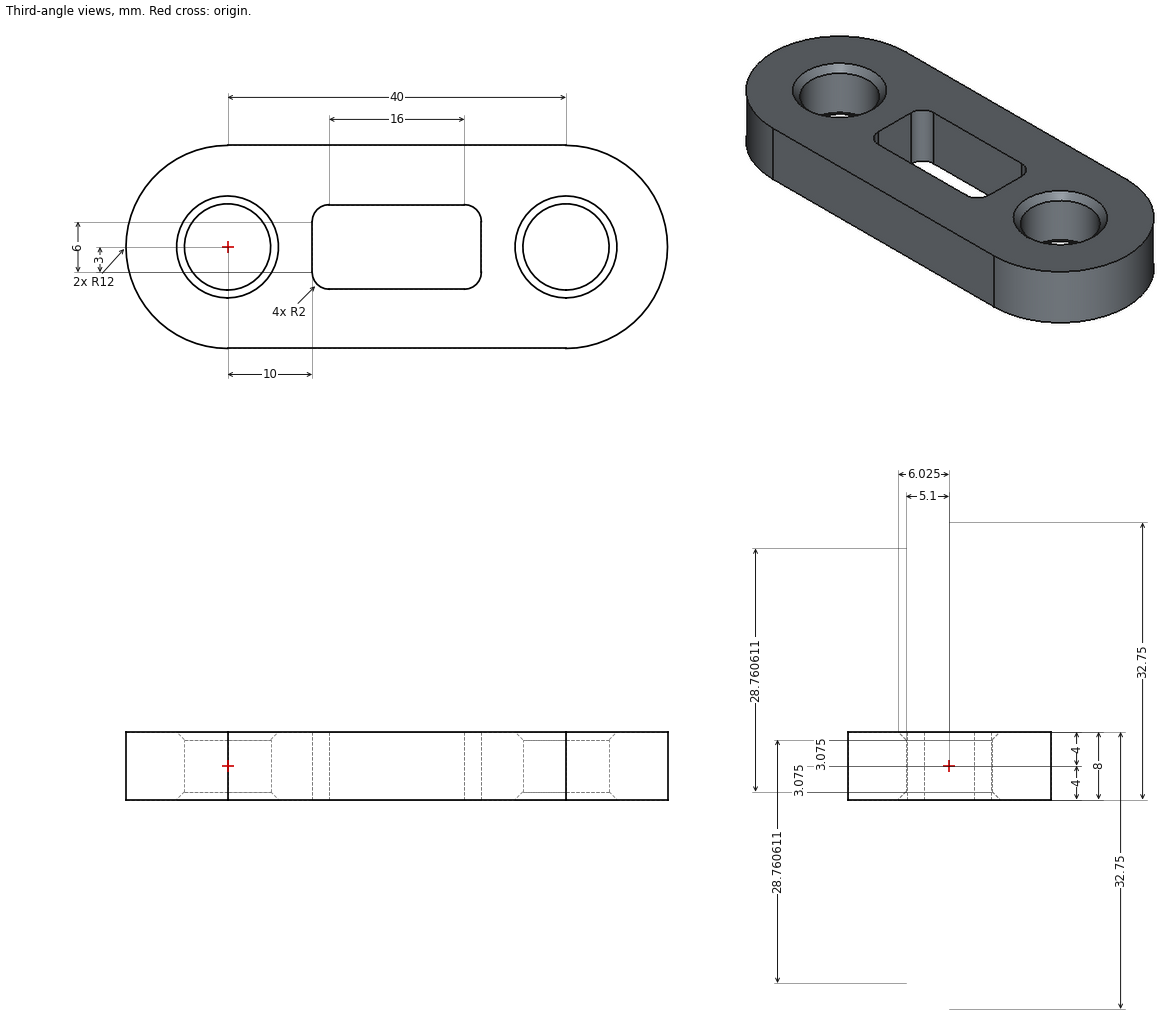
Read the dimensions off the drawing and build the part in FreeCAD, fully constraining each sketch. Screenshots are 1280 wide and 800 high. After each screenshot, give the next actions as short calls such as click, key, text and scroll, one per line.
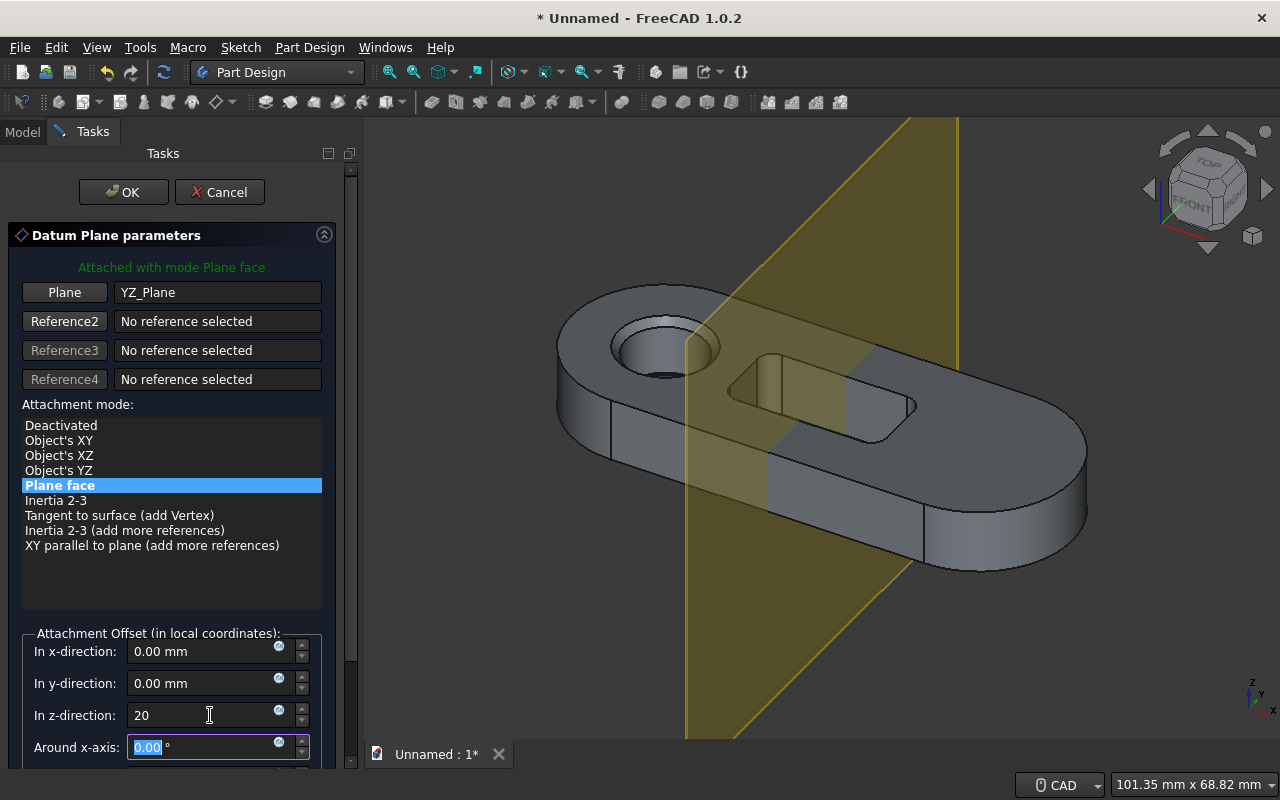
click(124, 192)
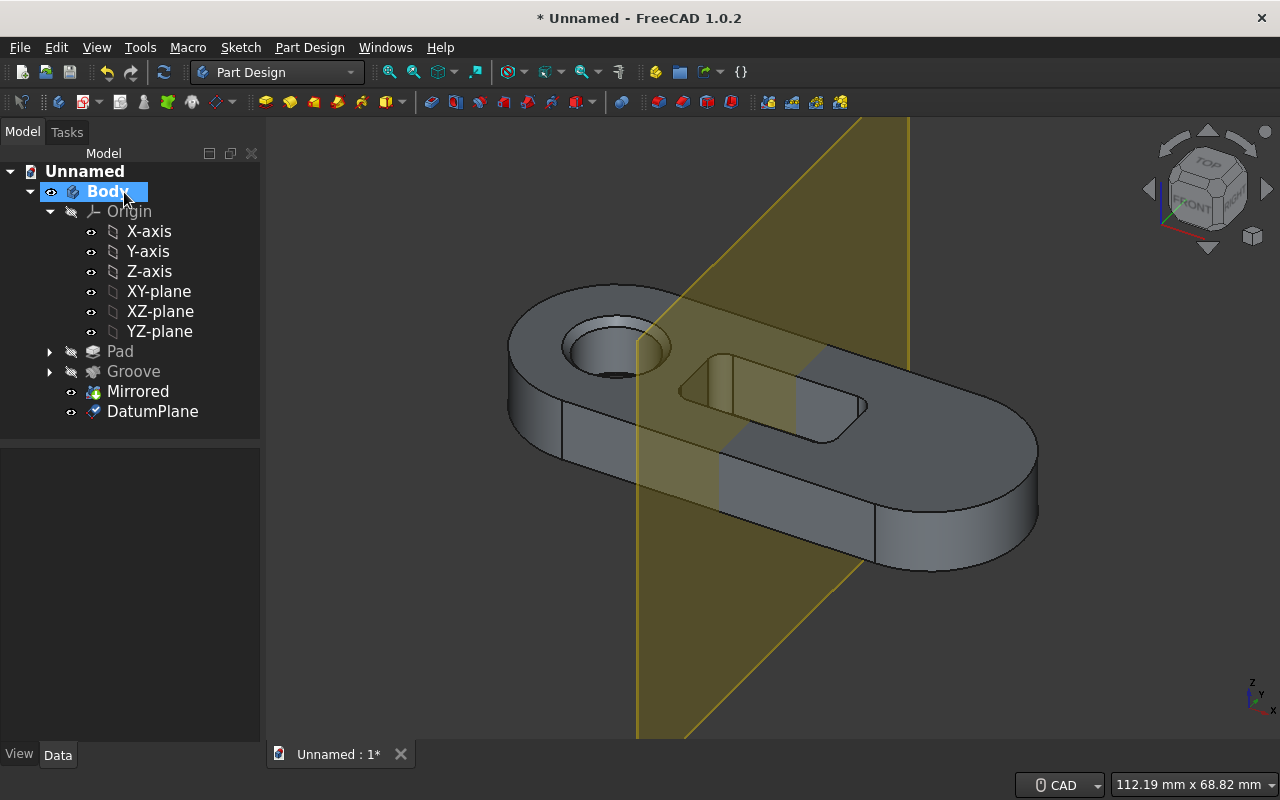
click(116, 372)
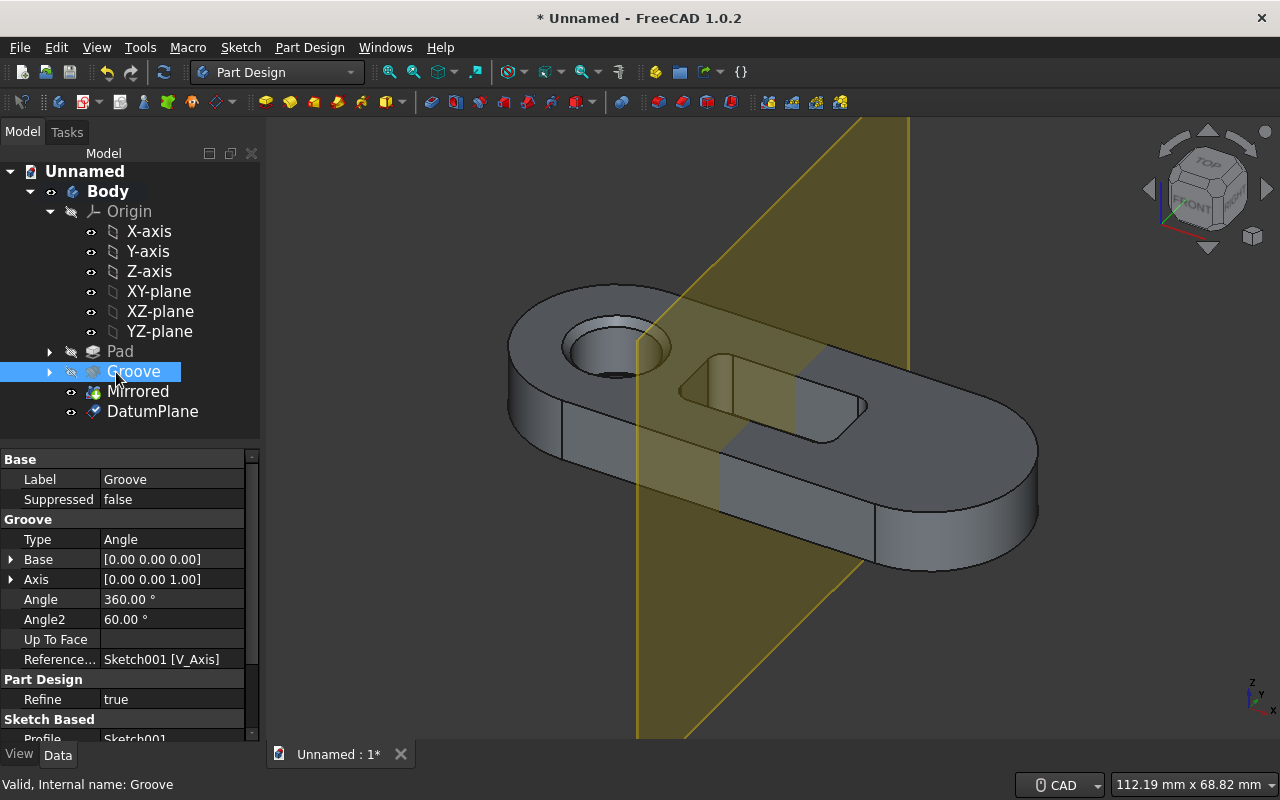
click(768, 102)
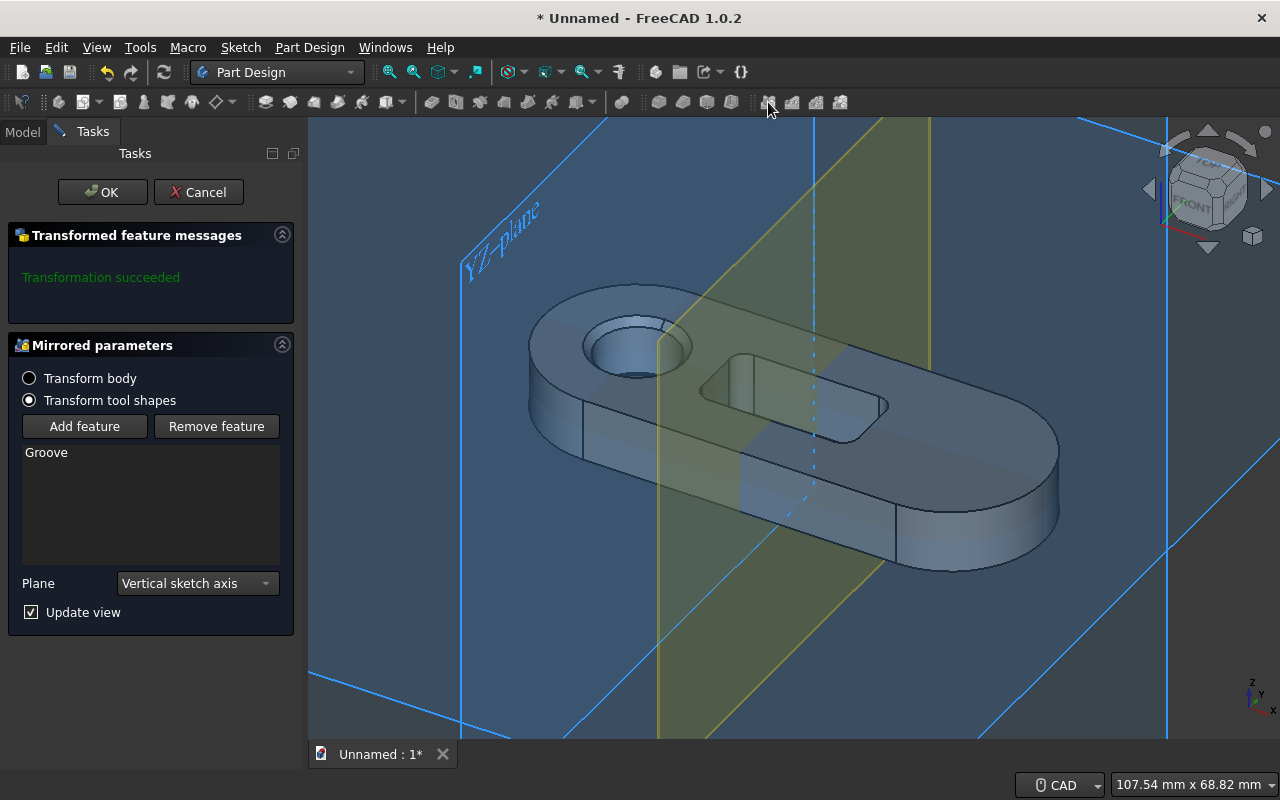
click(198, 584)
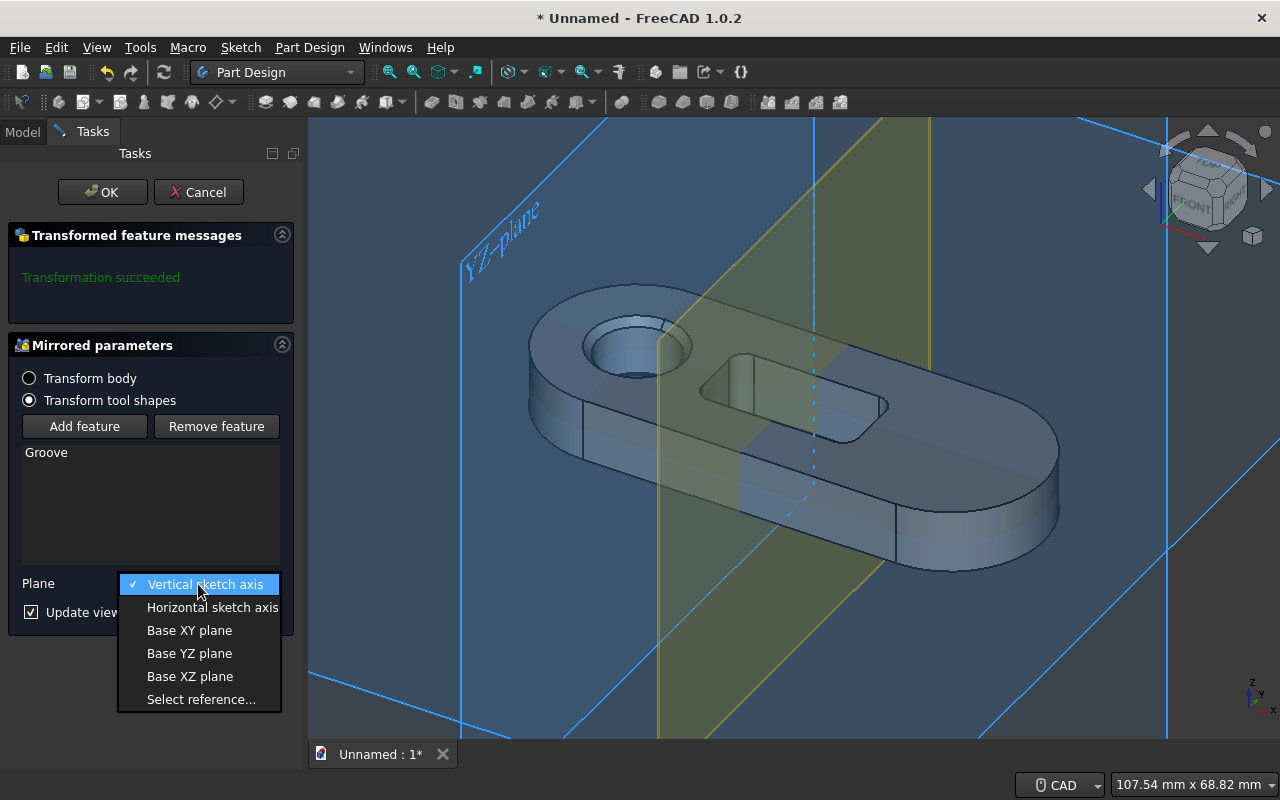
click(198, 700)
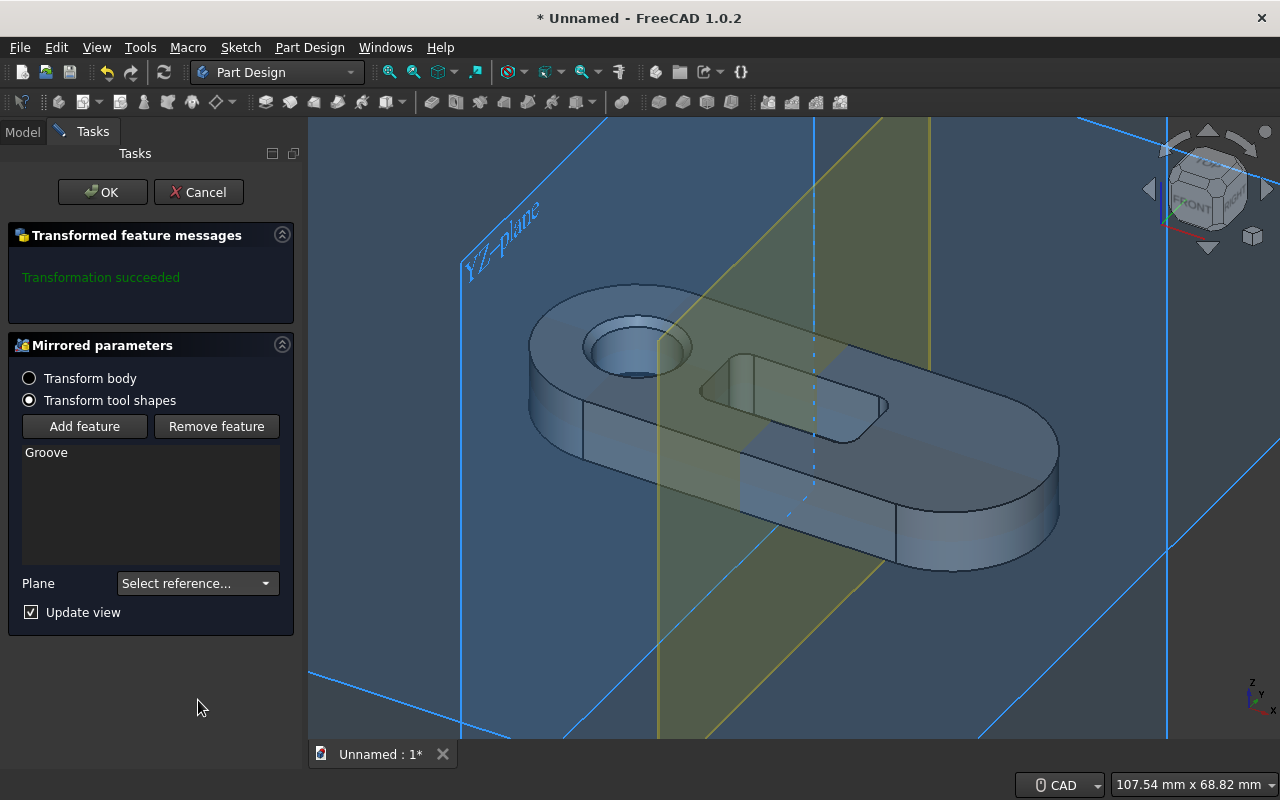
click(23, 131)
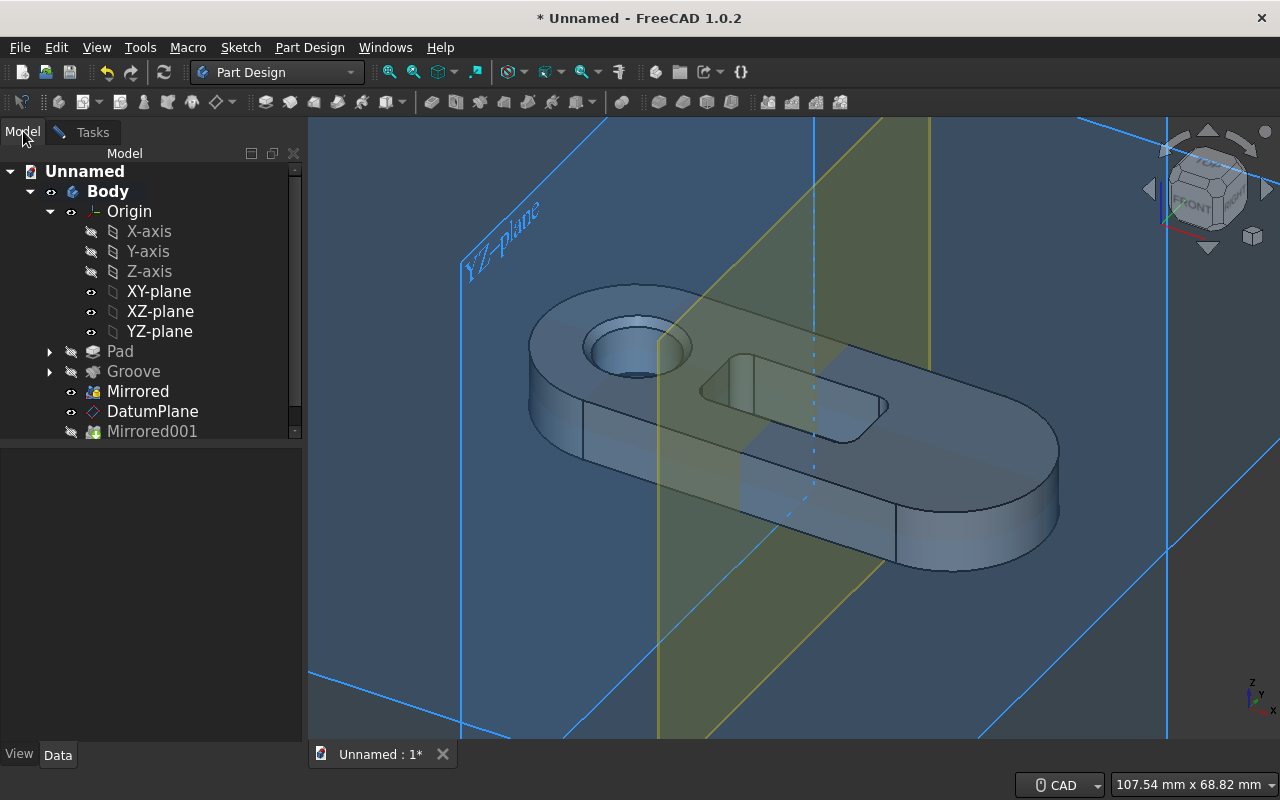
click(116, 412)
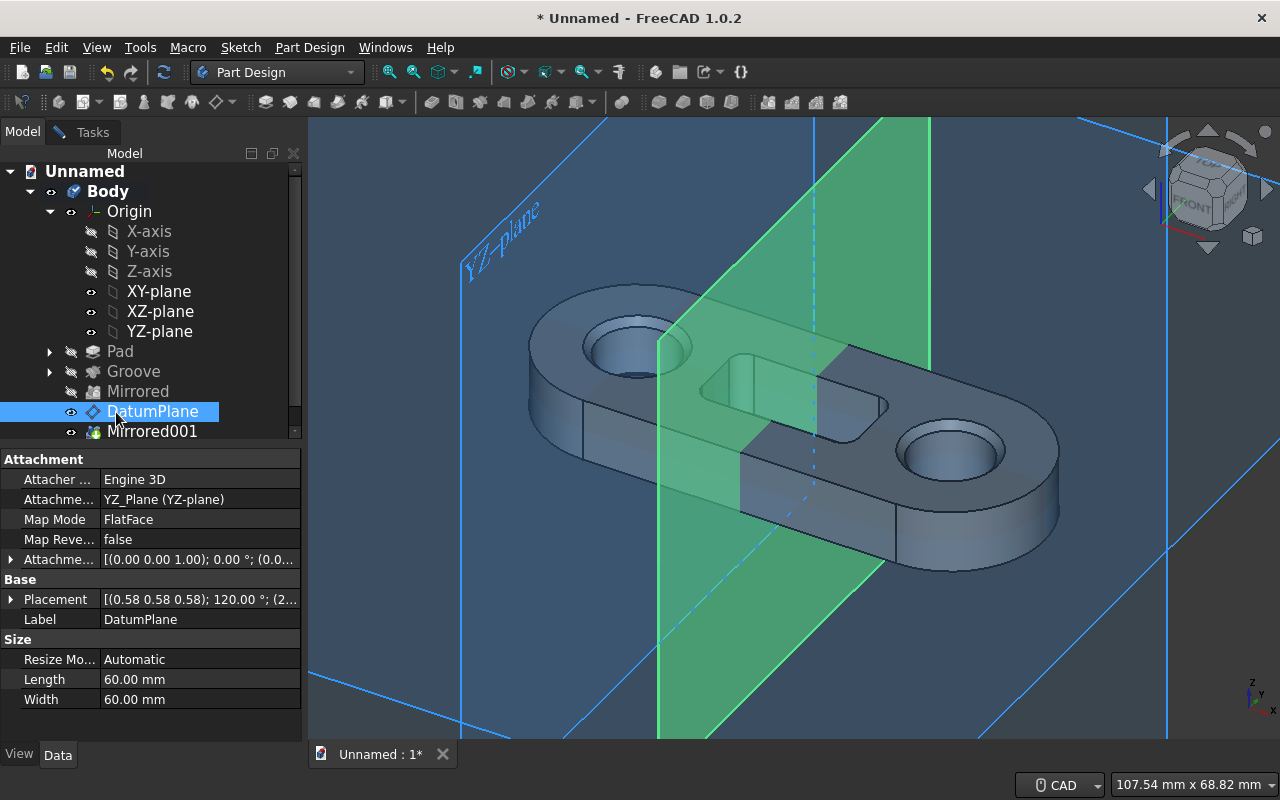
click(84, 131)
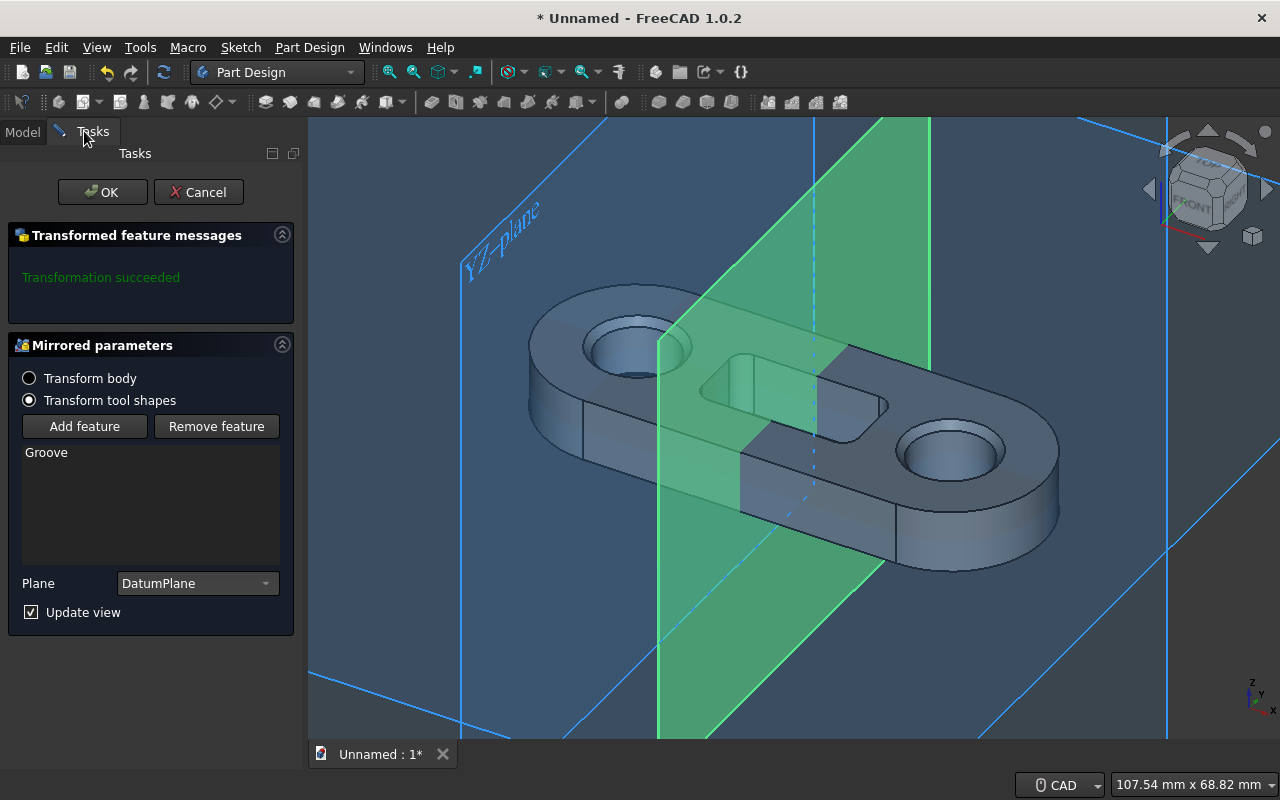
click(103, 192)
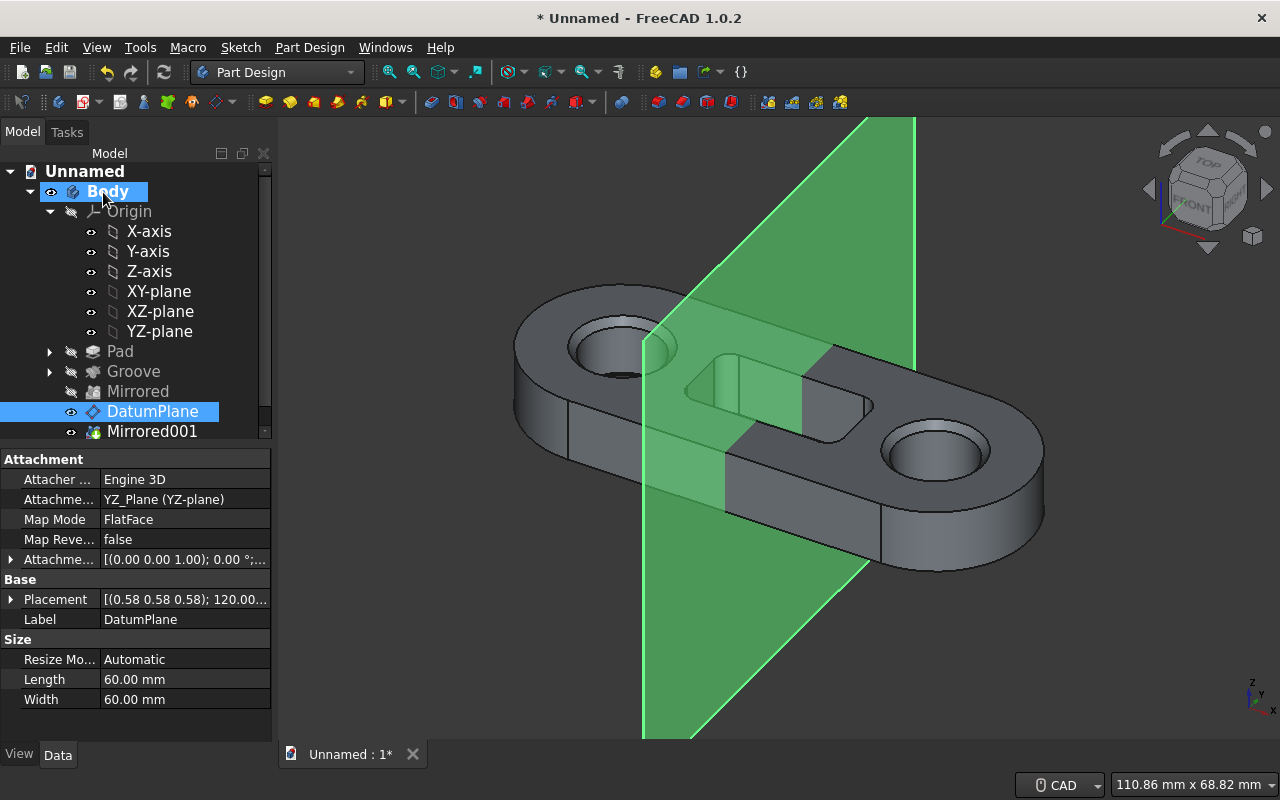
click(116, 412)
key(space)